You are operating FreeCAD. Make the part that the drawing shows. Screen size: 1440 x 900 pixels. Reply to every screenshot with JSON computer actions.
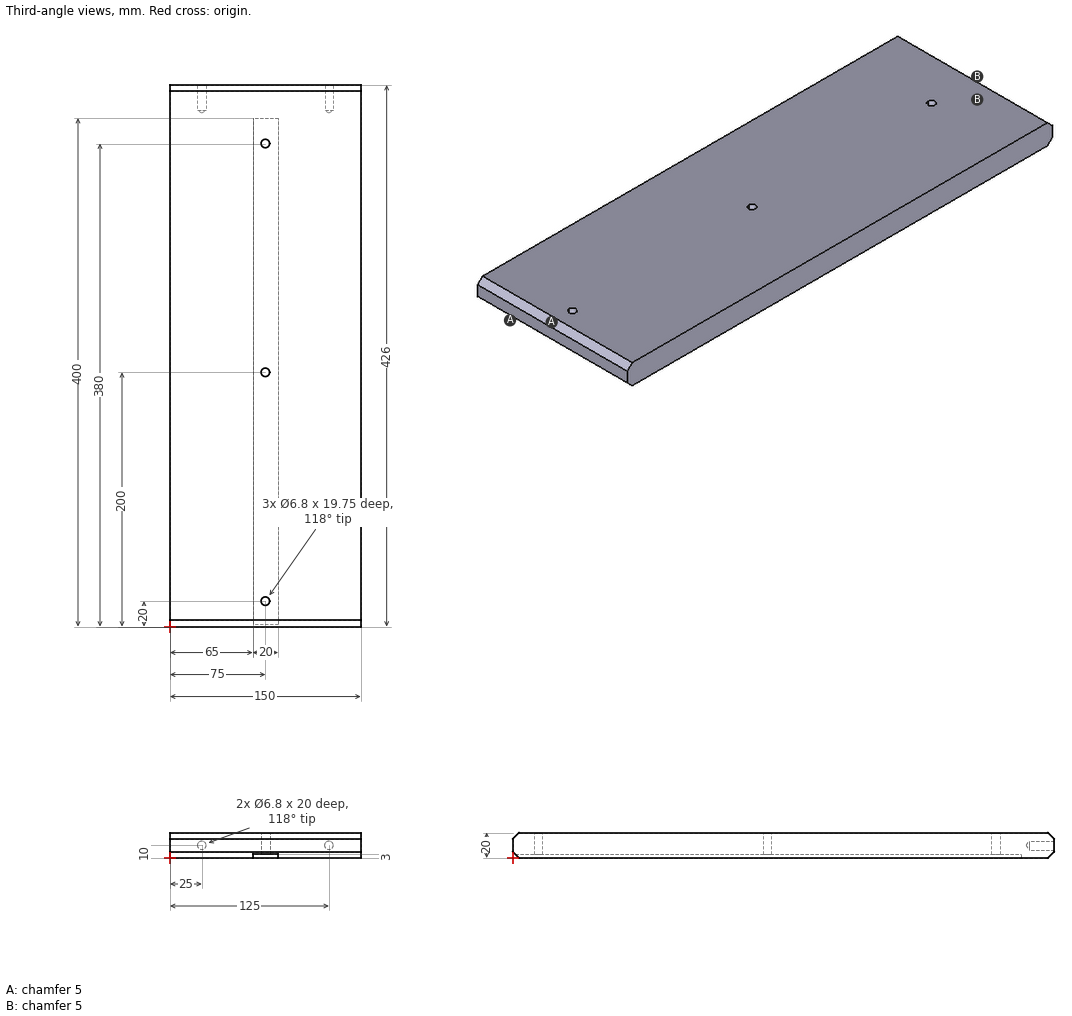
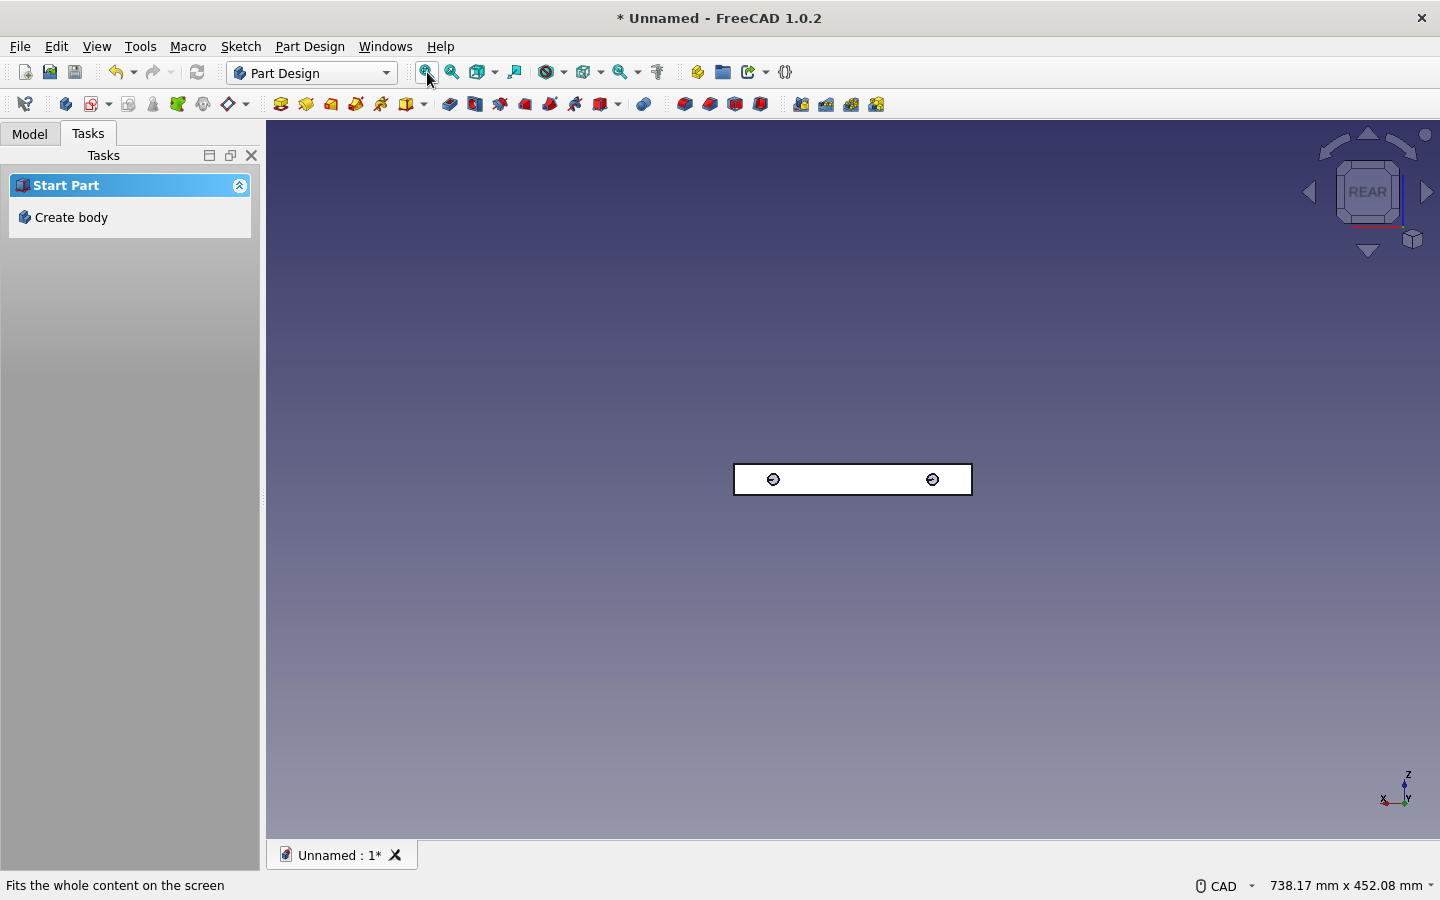
{"action": "left_click", "coordinate": [853, 463]}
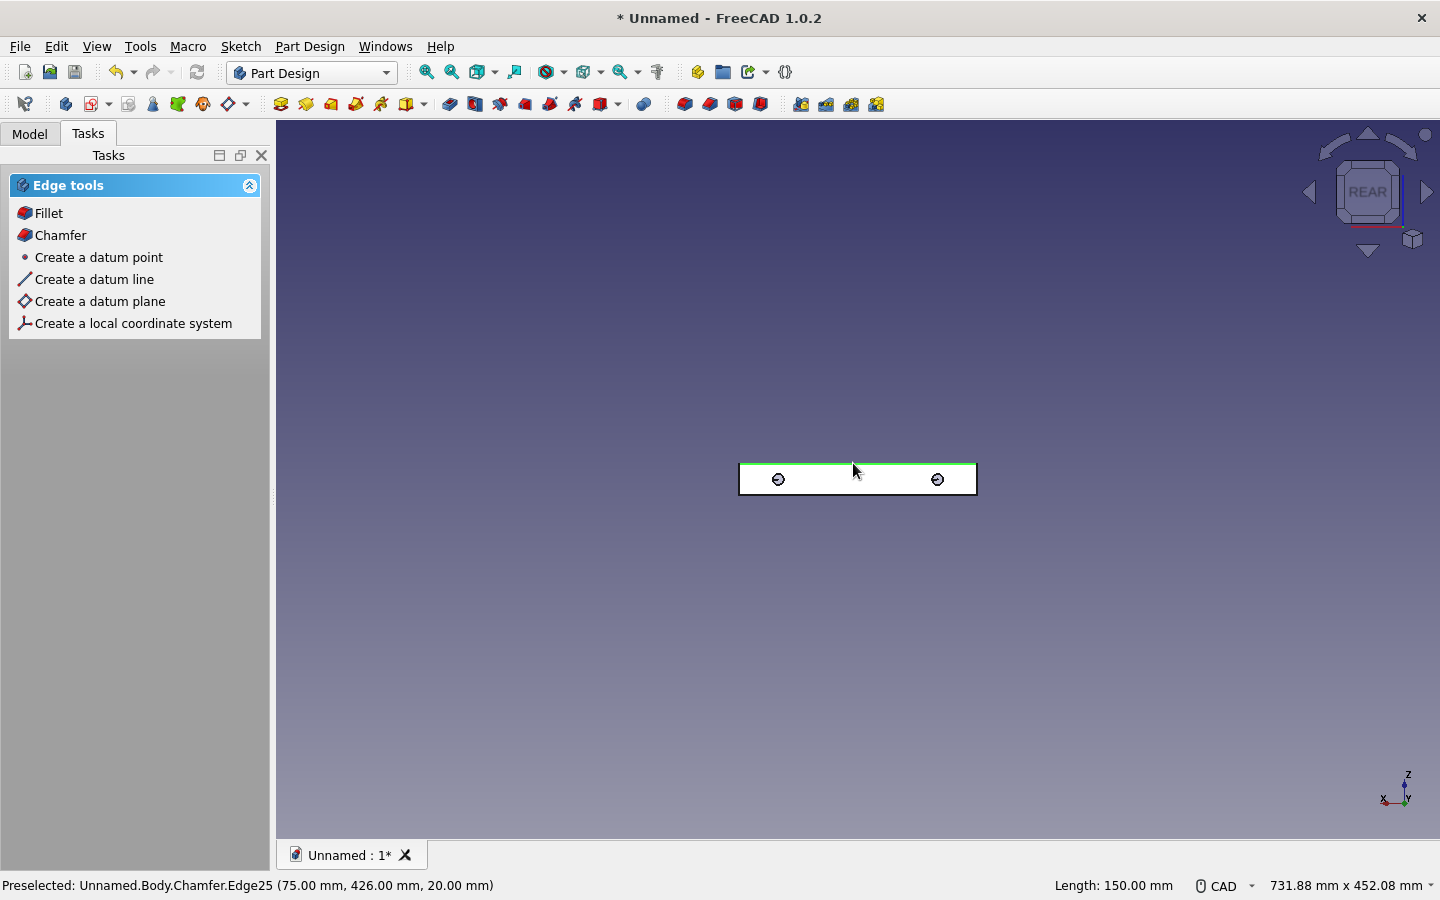
{"action": "left_click", "coordinate": [858, 494], "text": "ctrl"}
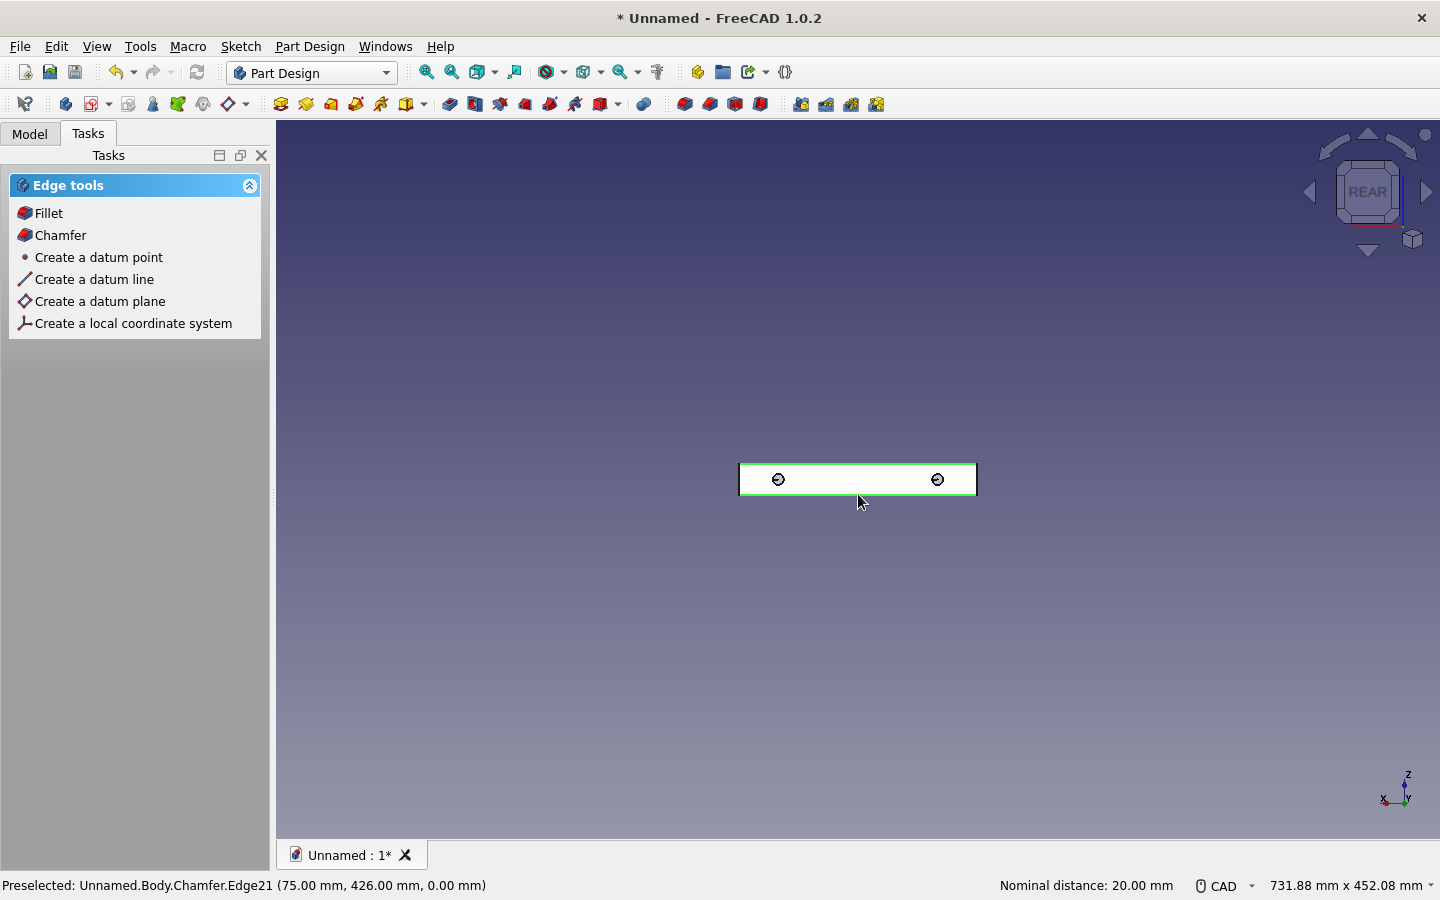
{"action": "left_click", "coordinate": [710, 104]}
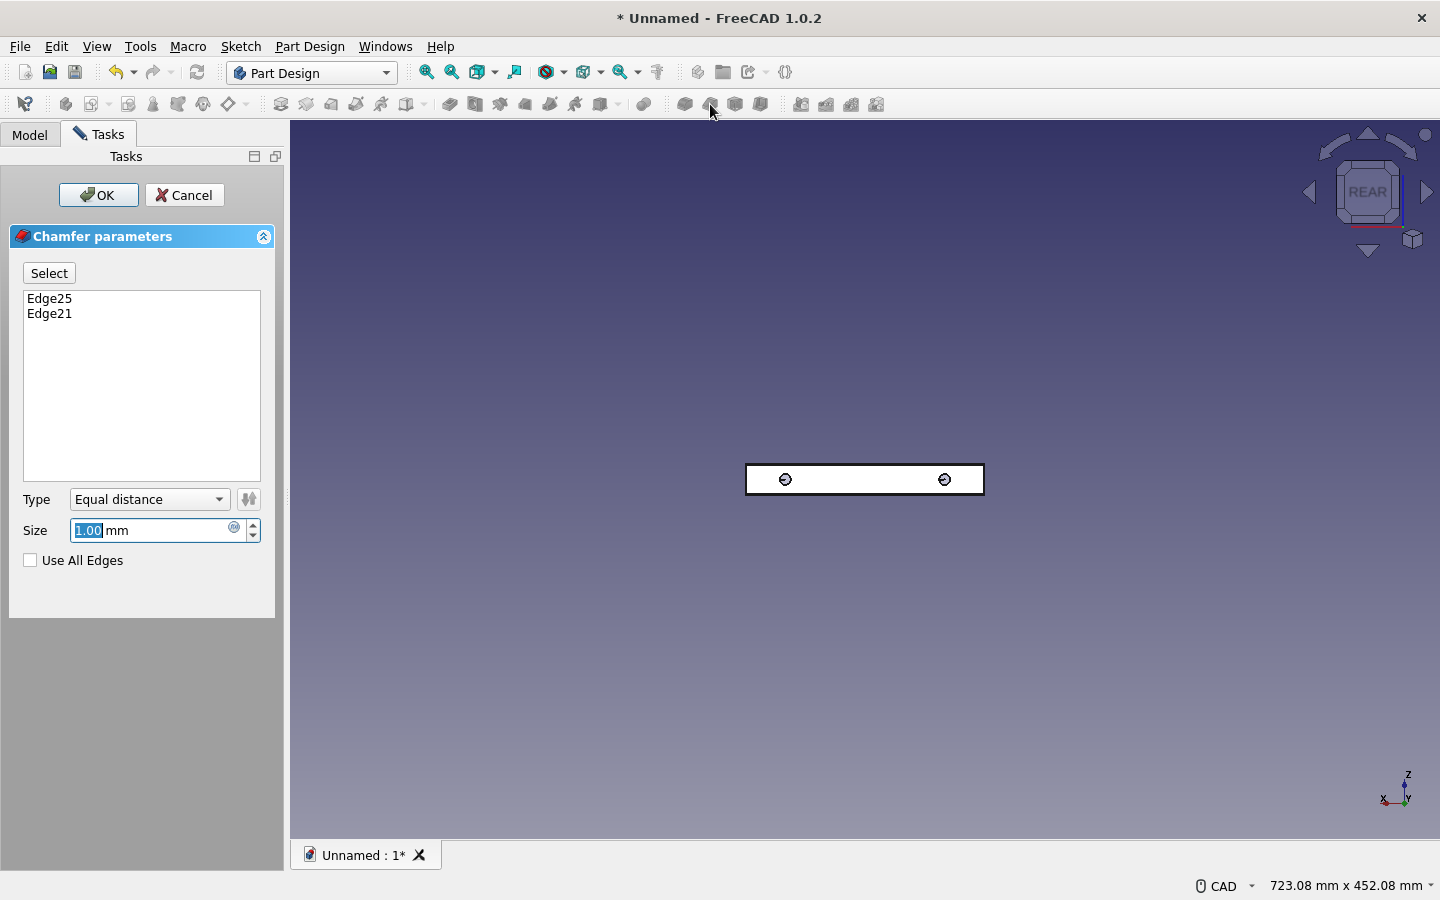
{"action": "type", "text": "5"}
{"action": "key", "text": "Tab"}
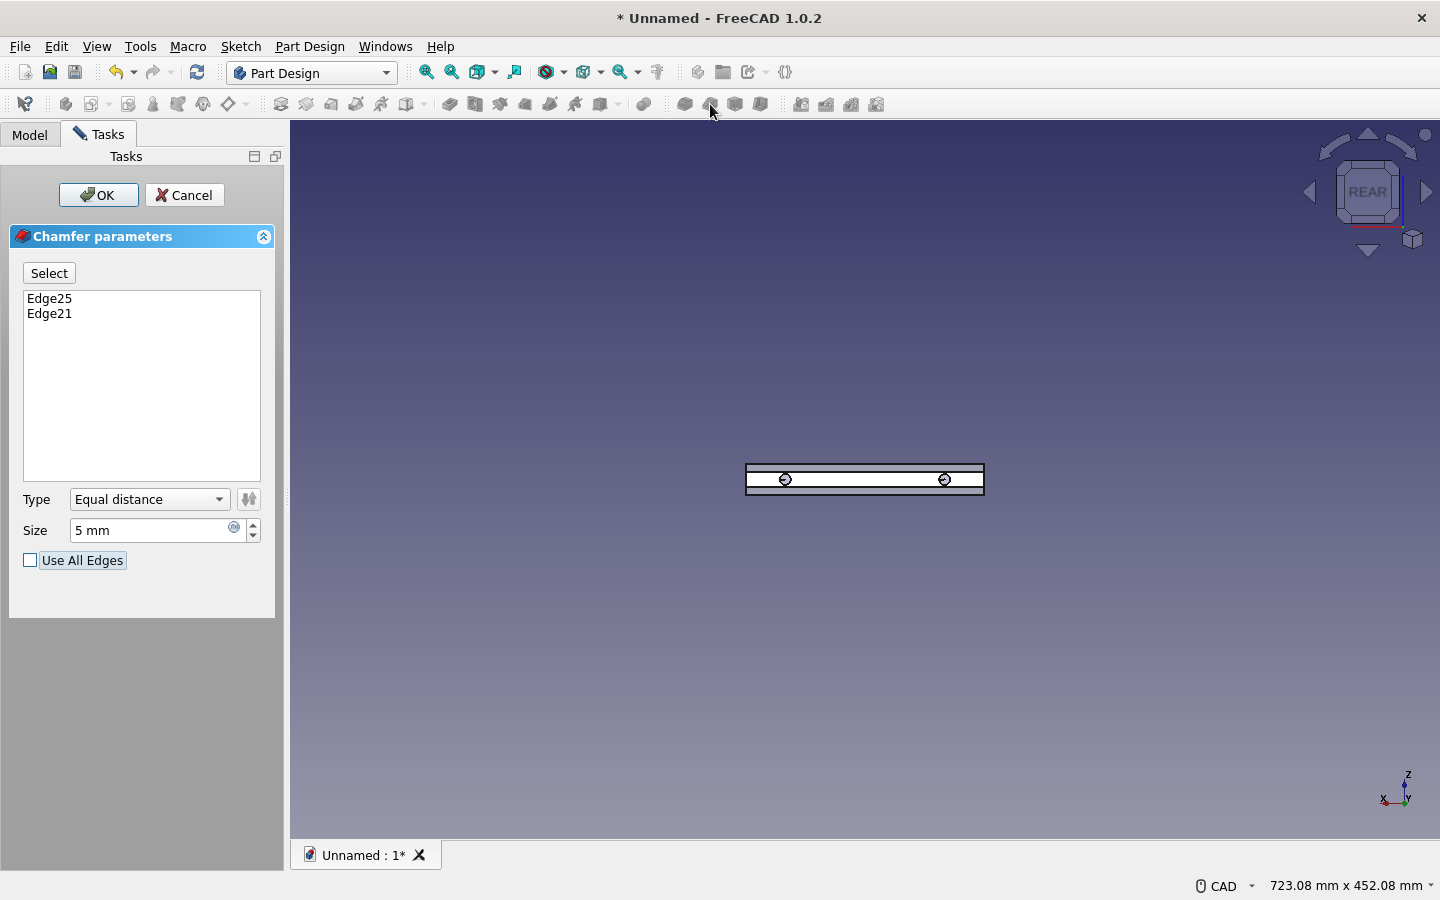
{"action": "left_click", "coordinate": [99, 195]}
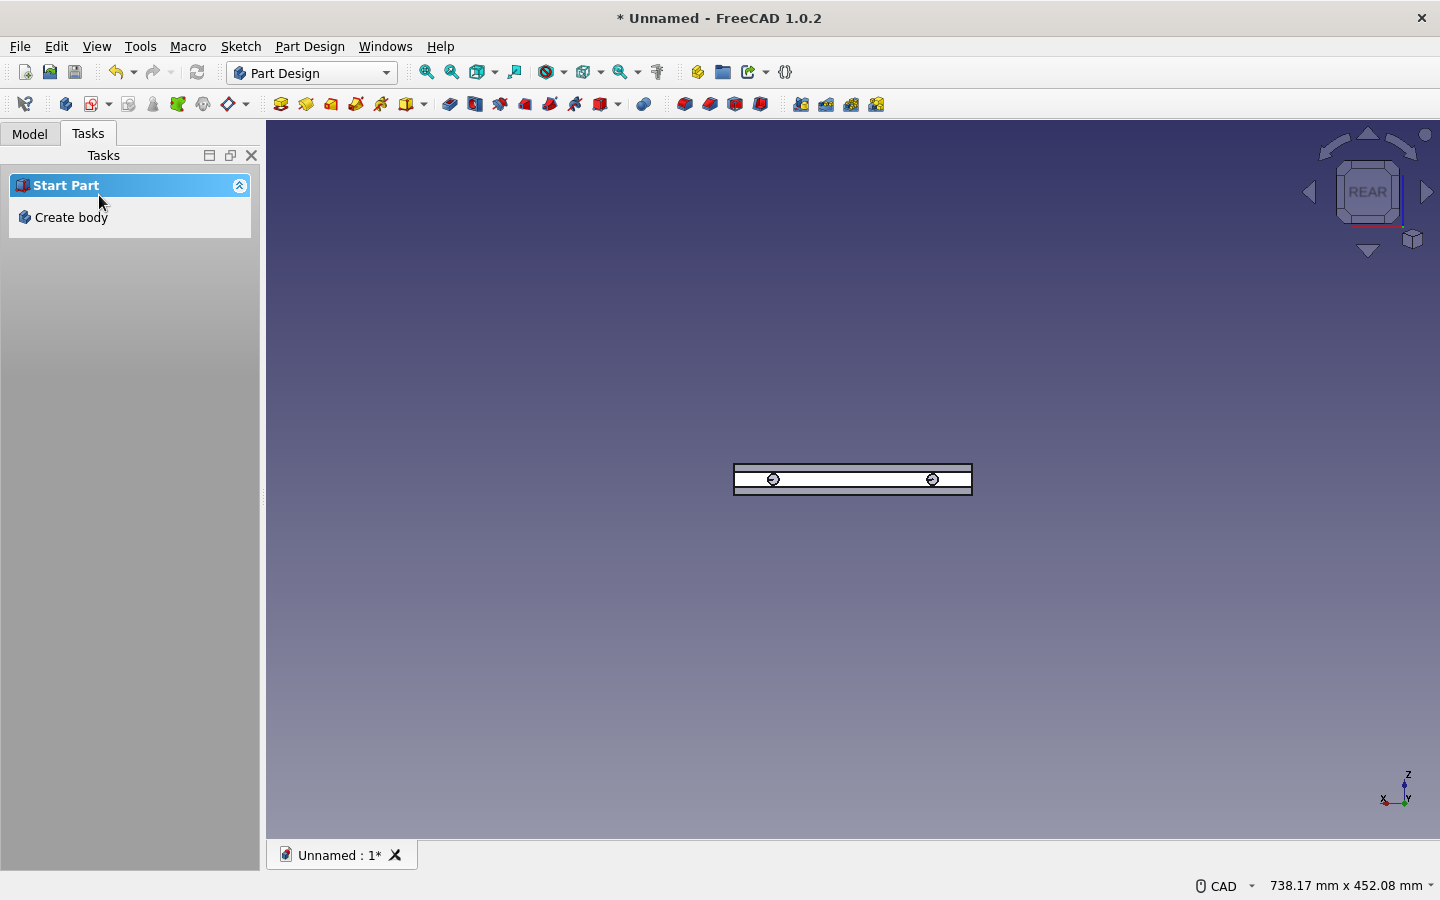
{"action": "key", "text": "0"}